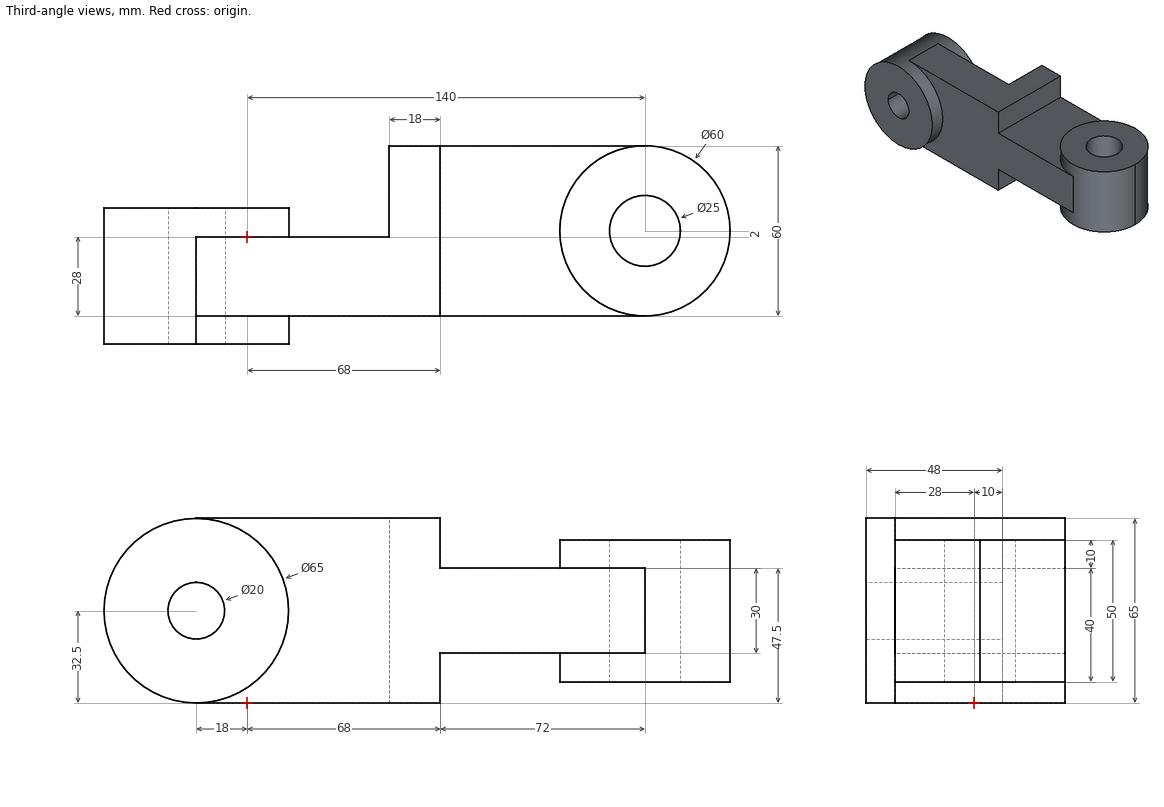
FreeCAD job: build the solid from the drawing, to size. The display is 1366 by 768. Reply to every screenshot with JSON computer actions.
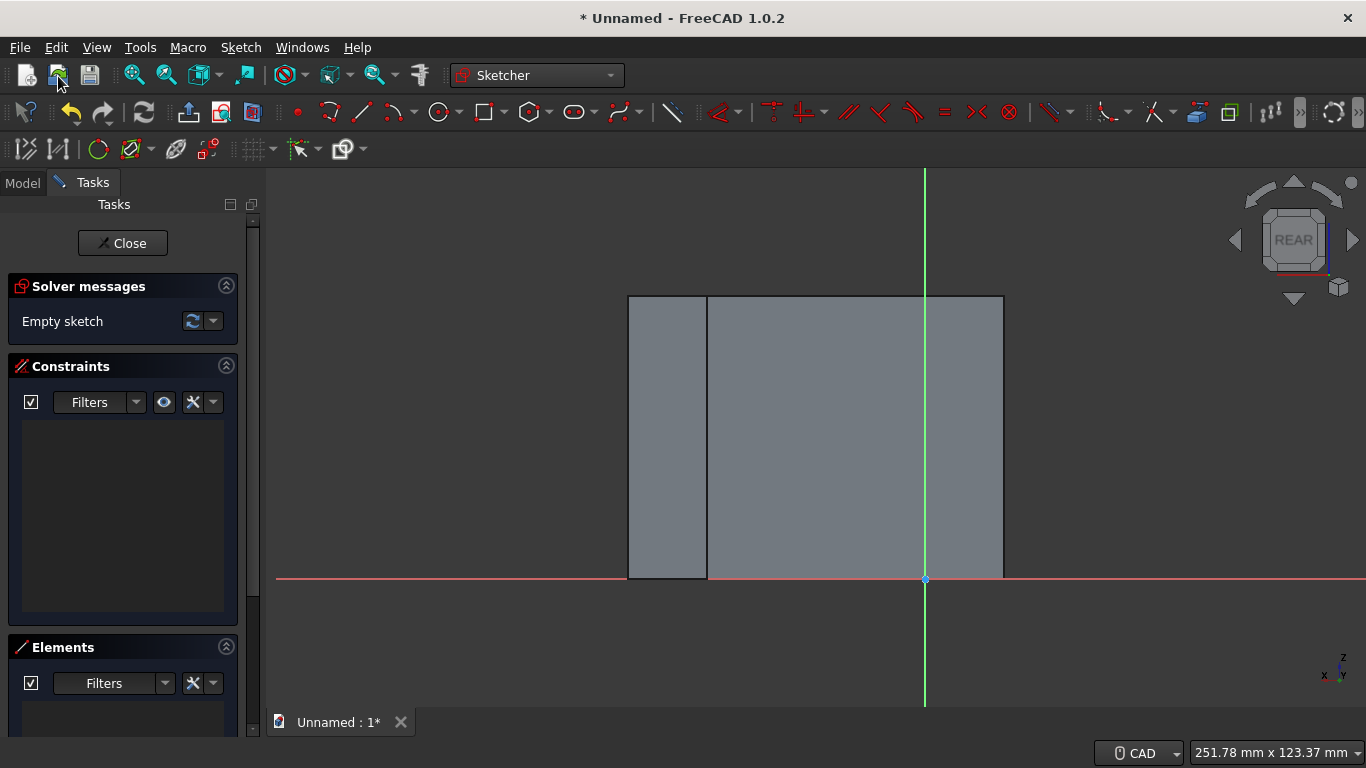
{"action": "key", "text": "q s"}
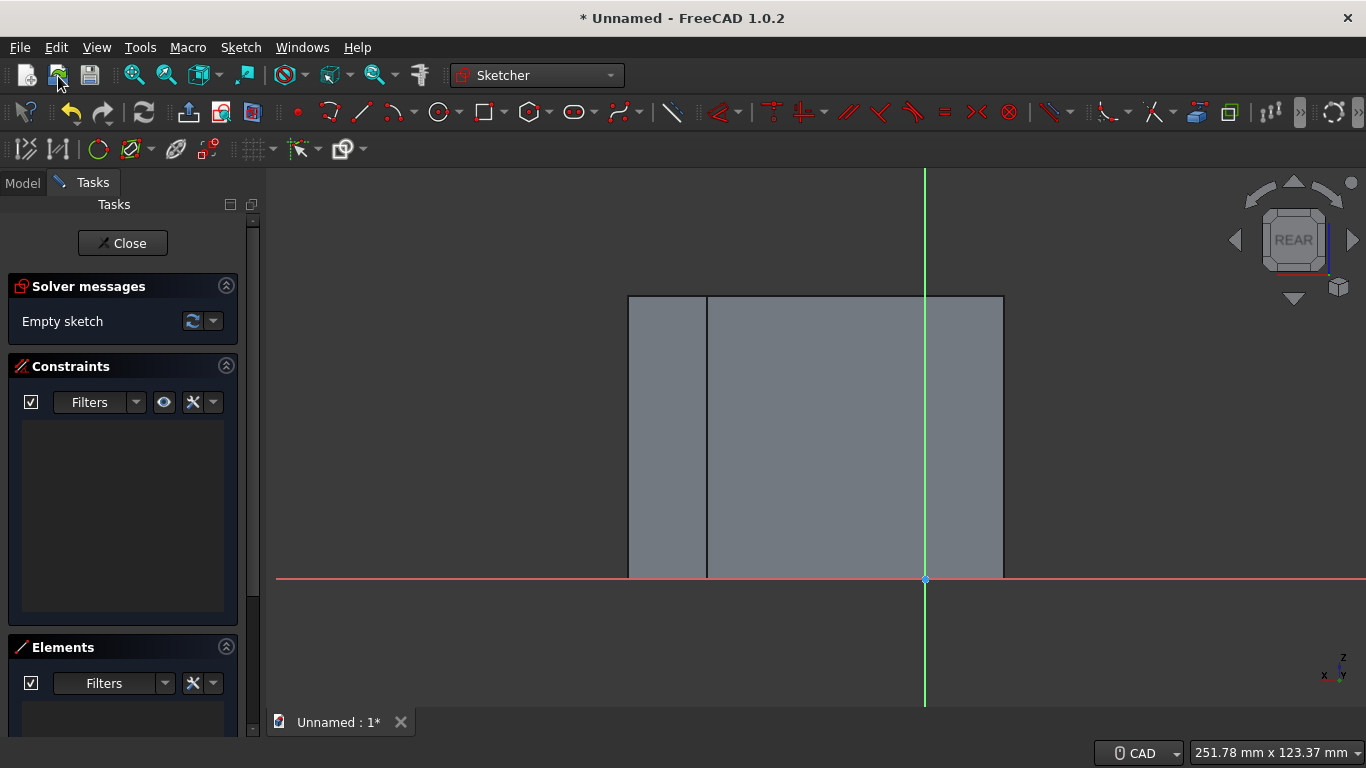
{"action": "left_click", "coordinate": [440, 112]}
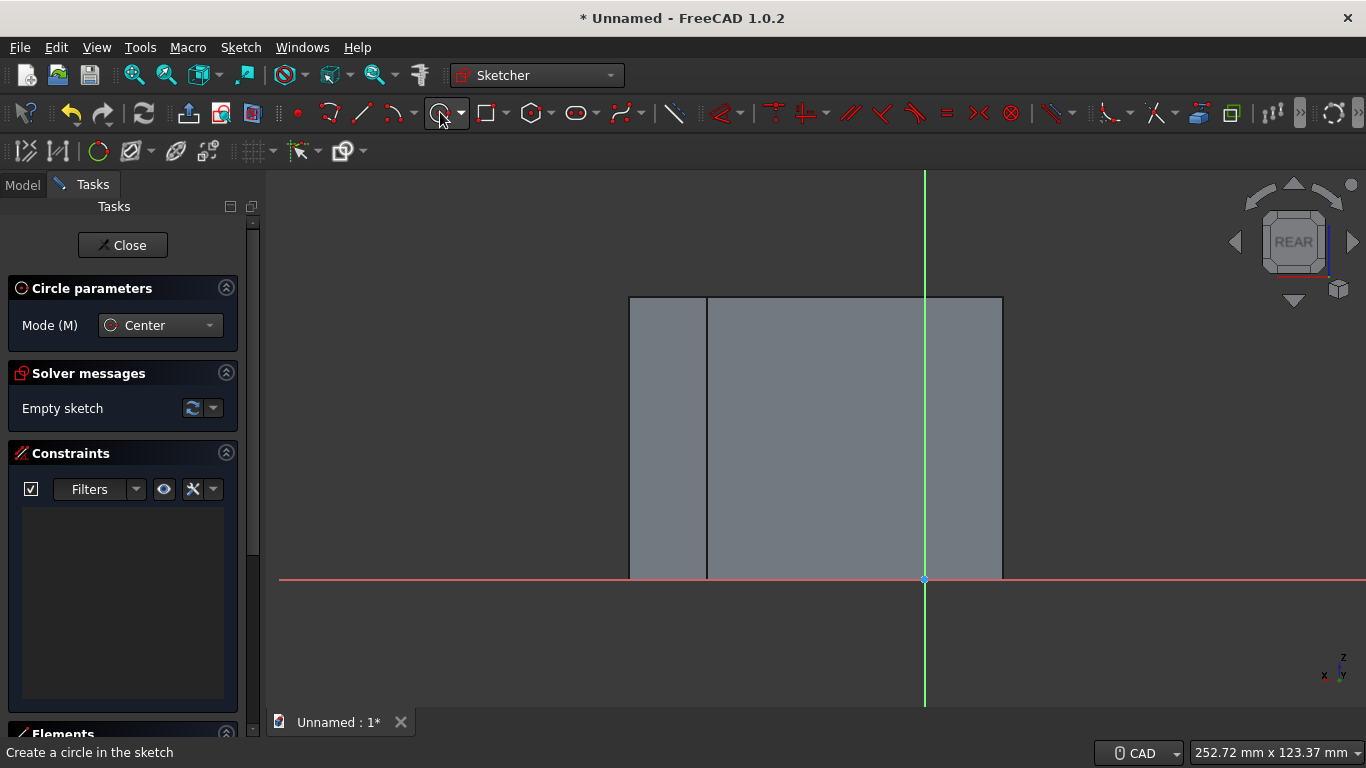
{"action": "left_click", "coordinate": [1003, 438]}
{"action": "left_click", "coordinate": [1103, 338]}
{"action": "key", "text": "Escape"}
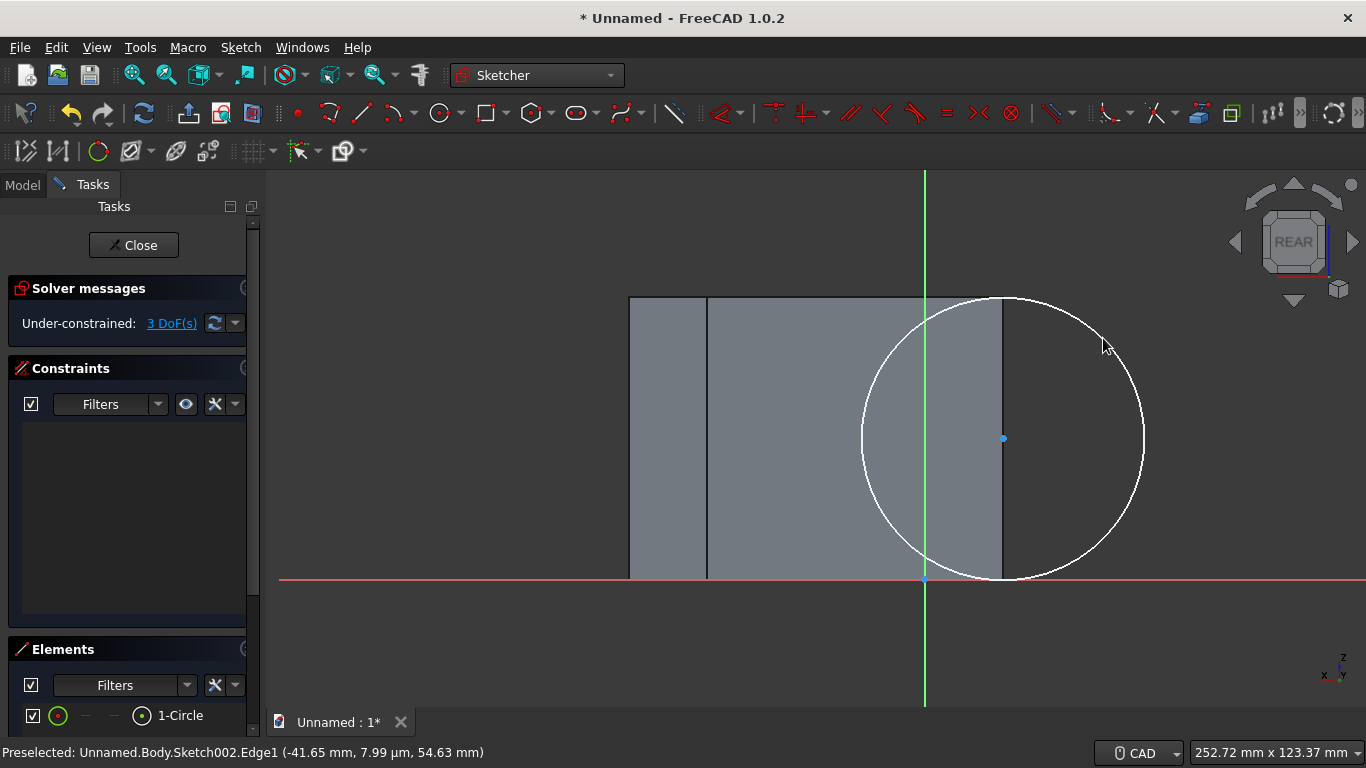
{"action": "left_click", "coordinate": [720, 114]}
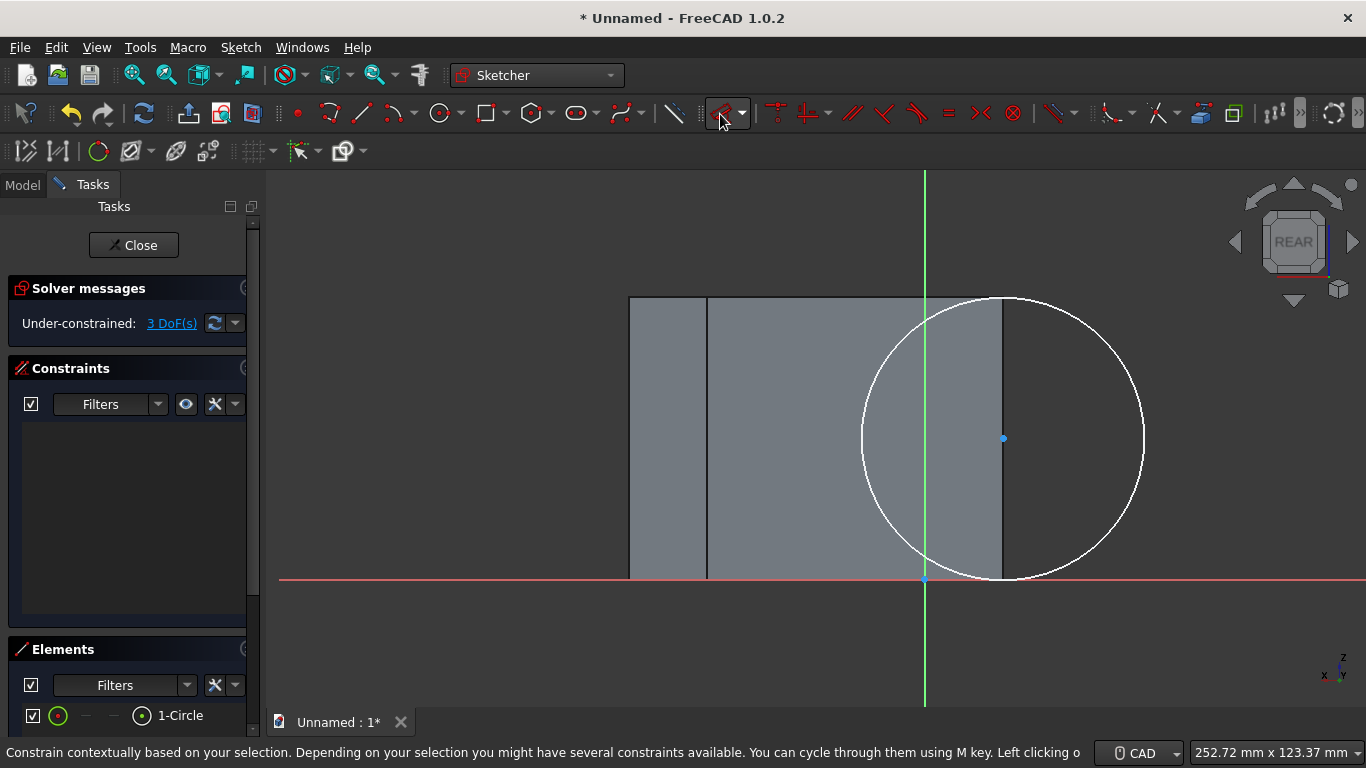
{"action": "left_click", "coordinate": [1103, 339]}
{"action": "left_click", "coordinate": [1126, 316]}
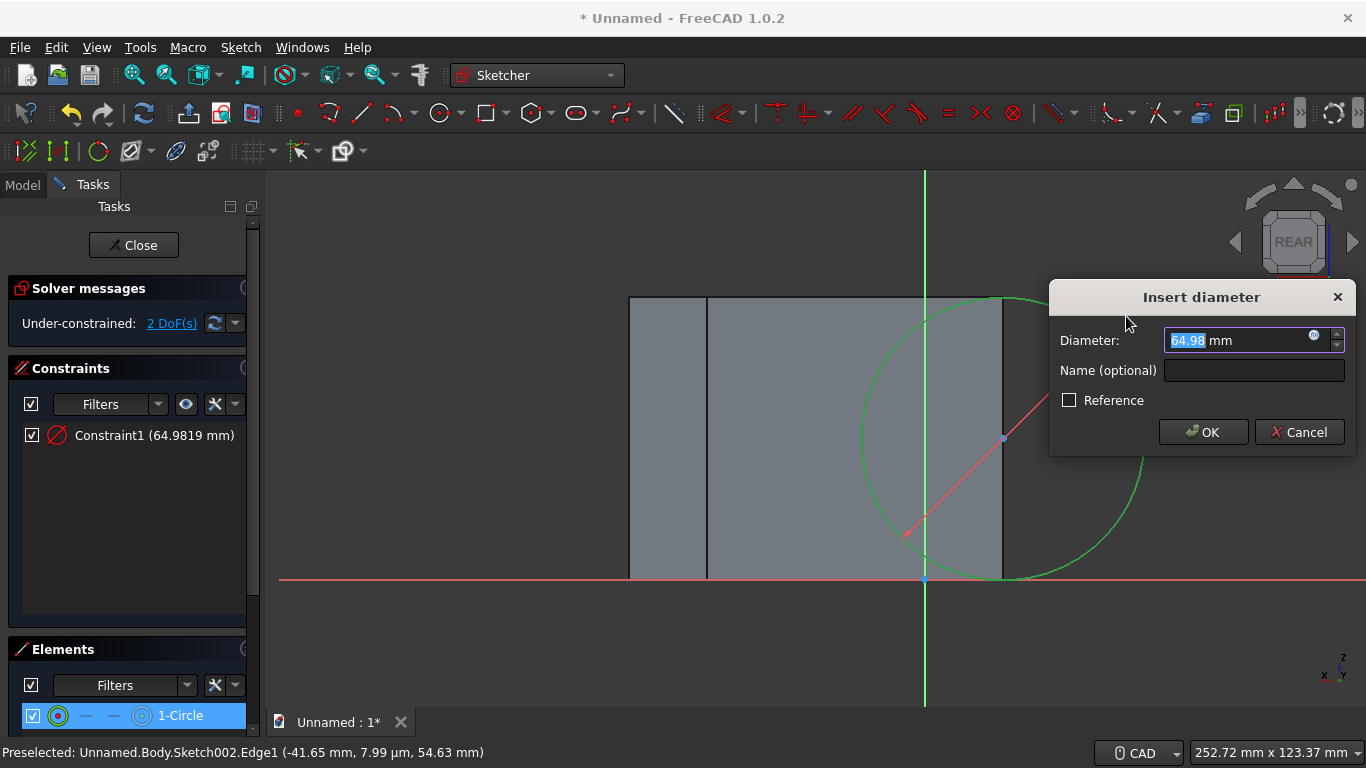
{"action": "type", "text": "65"}
{"action": "key", "text": "Return"}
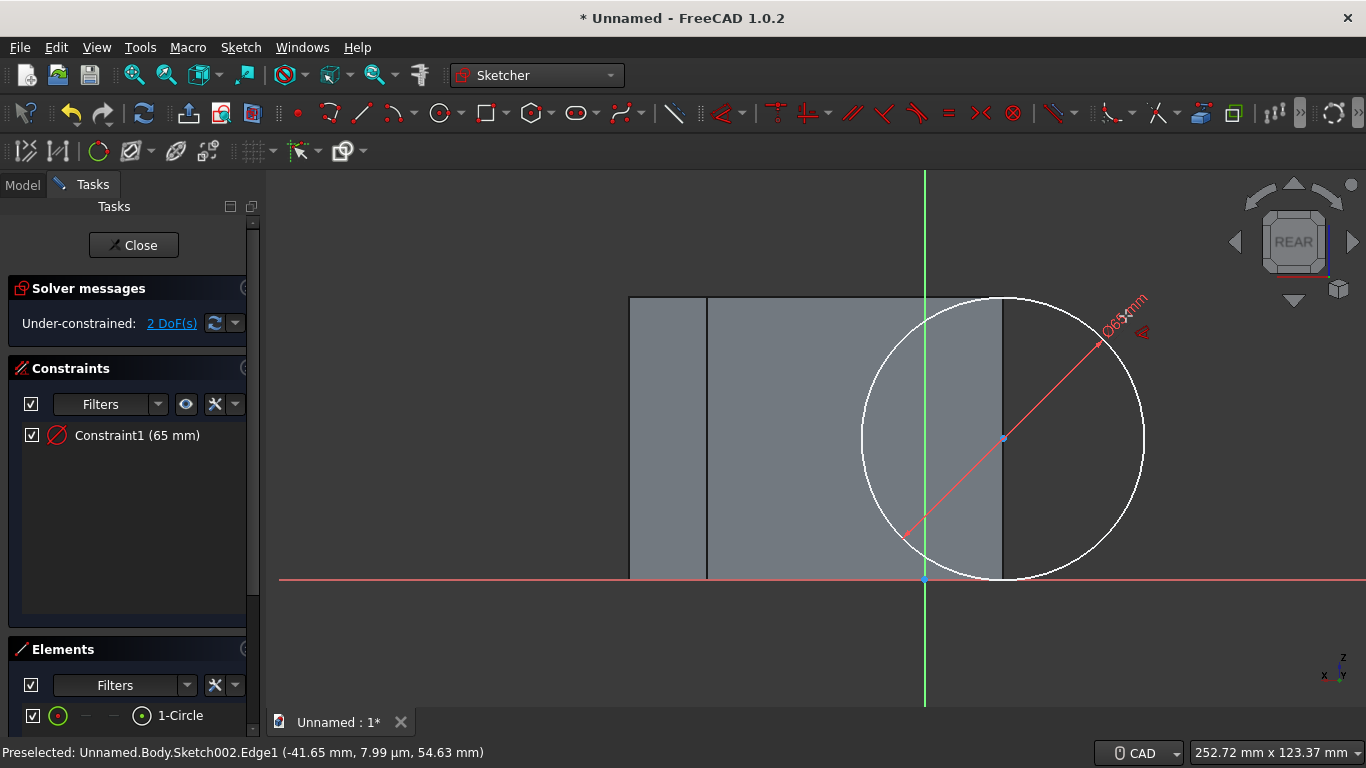
{"action": "left_click", "coordinate": [1003, 439]}
{"action": "left_click", "coordinate": [964, 614]}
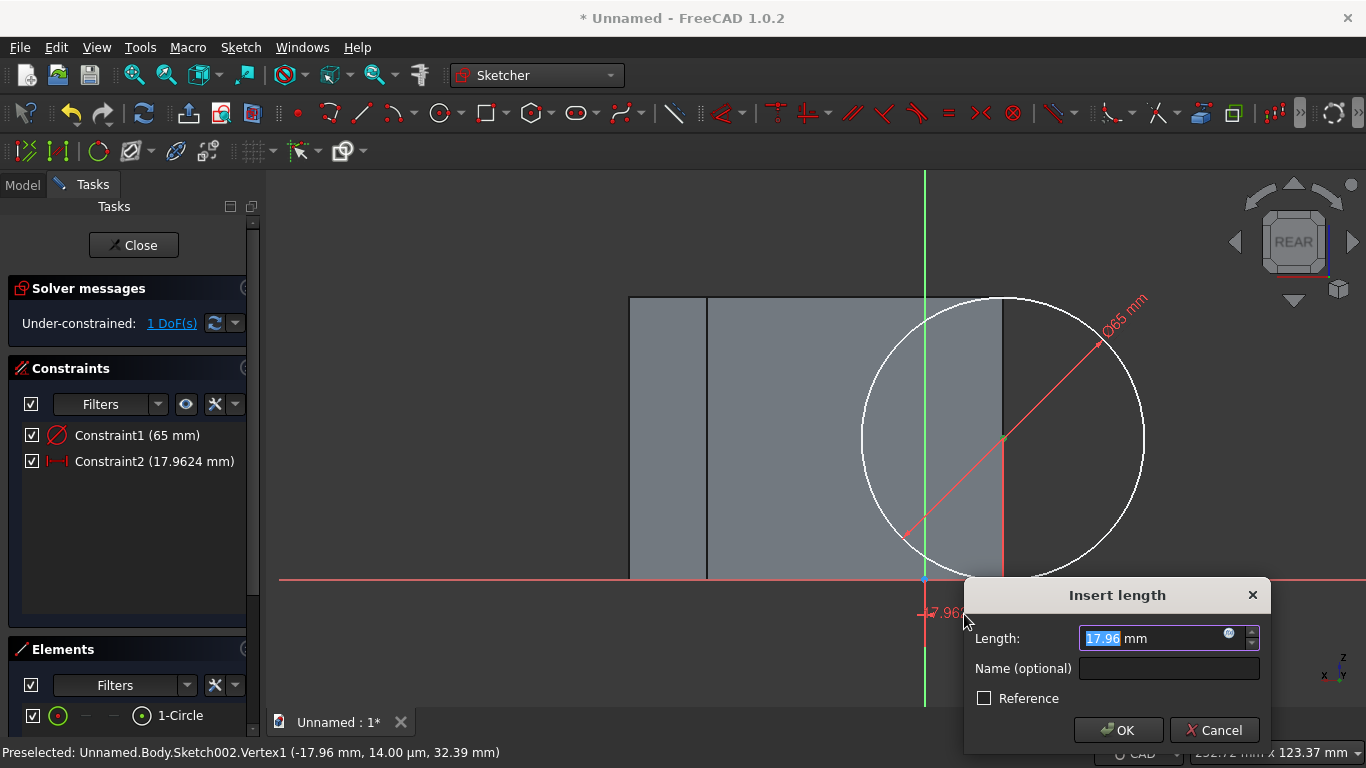
{"action": "type", "text": "18"}
{"action": "key", "text": "Return"}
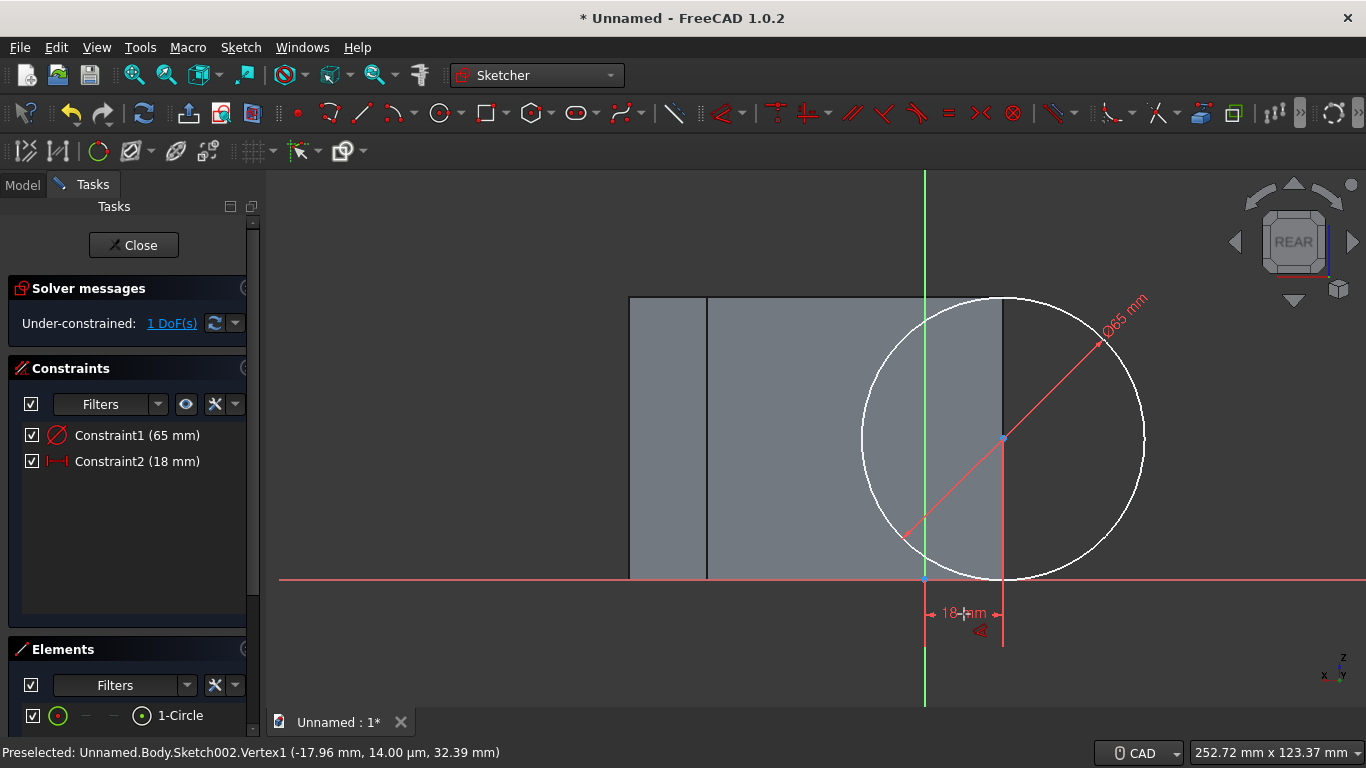
{"action": "left_click", "coordinate": [1003, 439]}
{"action": "left_click", "coordinate": [891, 477]}